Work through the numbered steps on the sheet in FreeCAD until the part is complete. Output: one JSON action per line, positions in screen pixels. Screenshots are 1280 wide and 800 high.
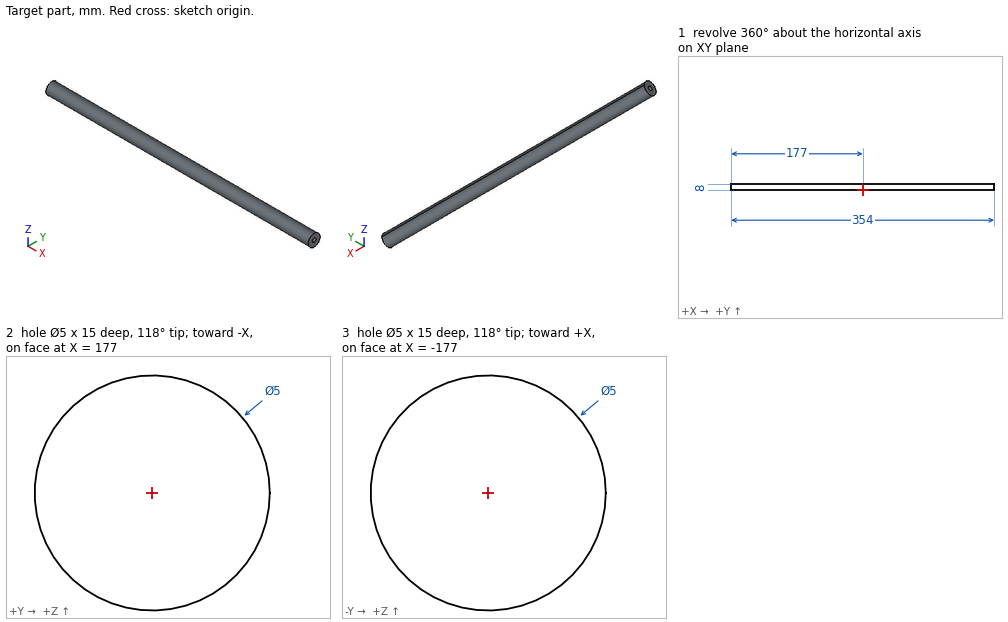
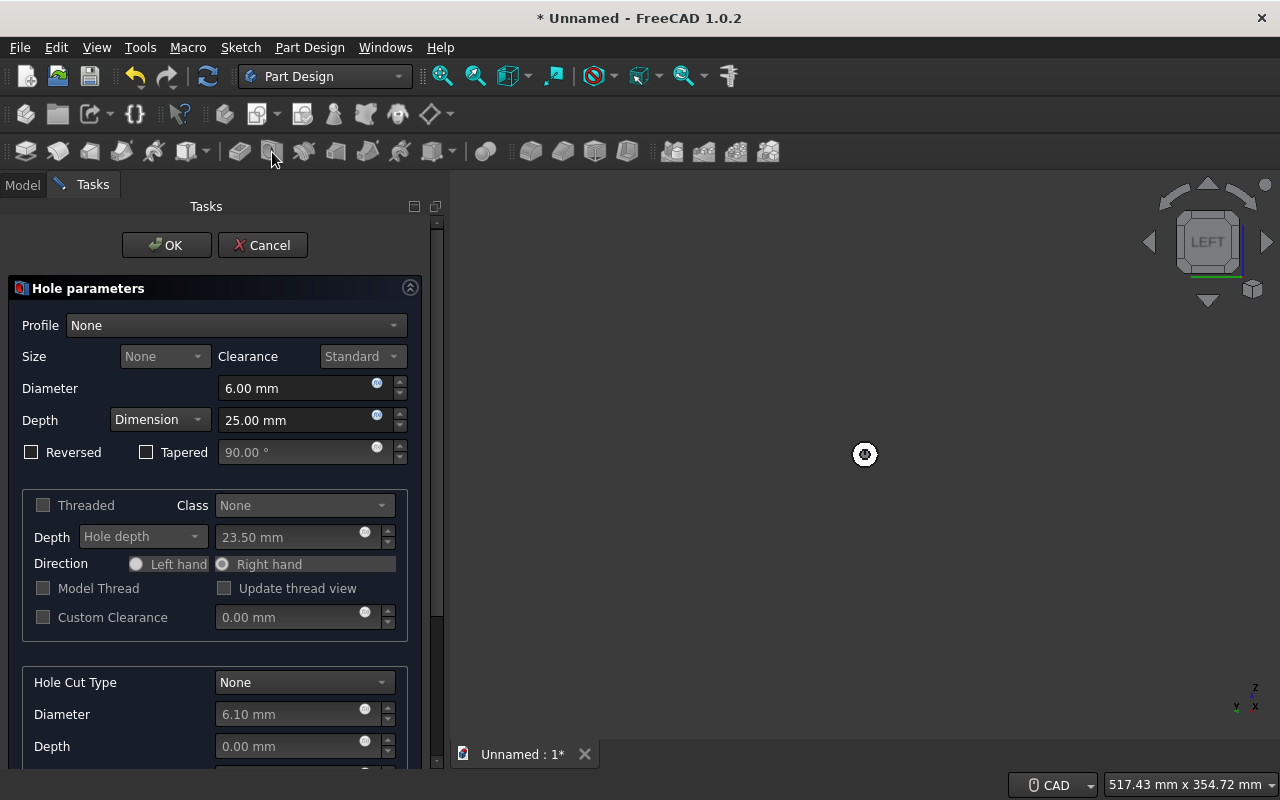
{"action": "triple_click", "coordinate": [305, 388]}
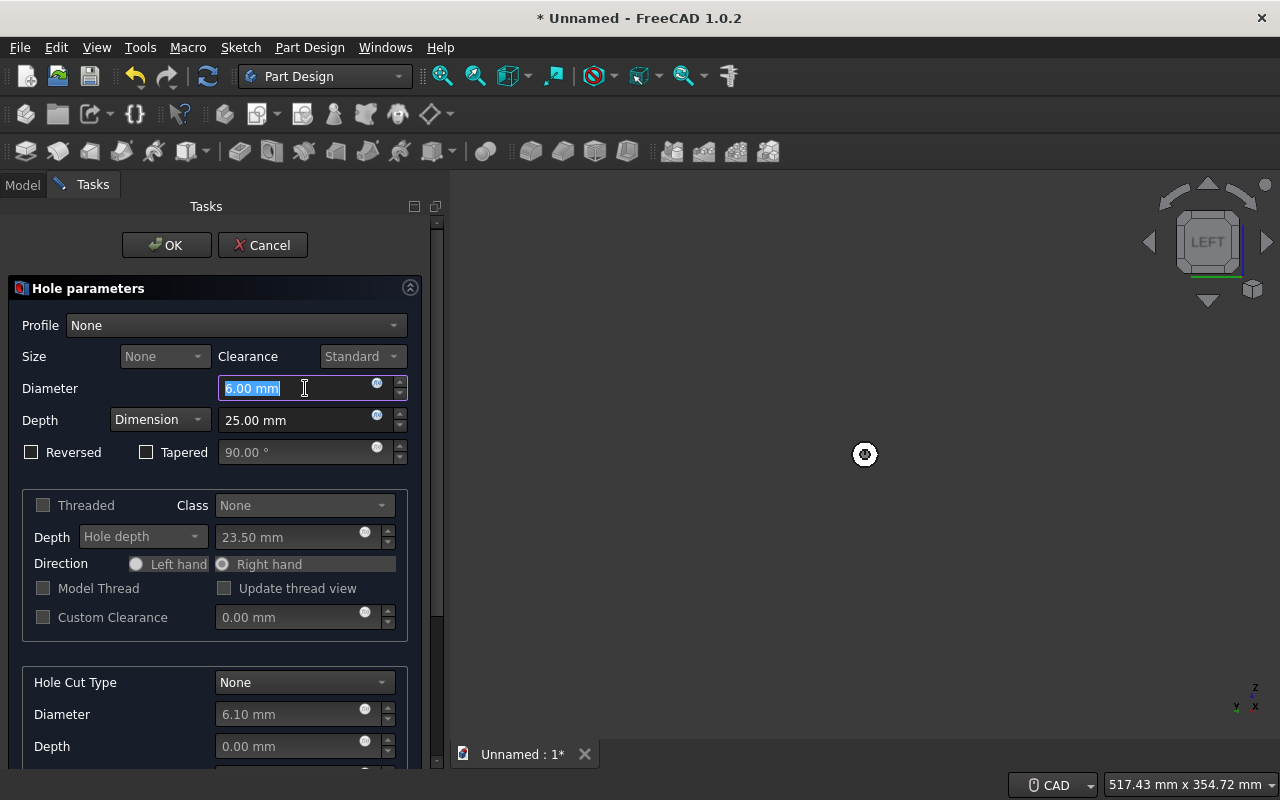
{"action": "type", "text": "5"}
{"action": "key", "text": "Tab"}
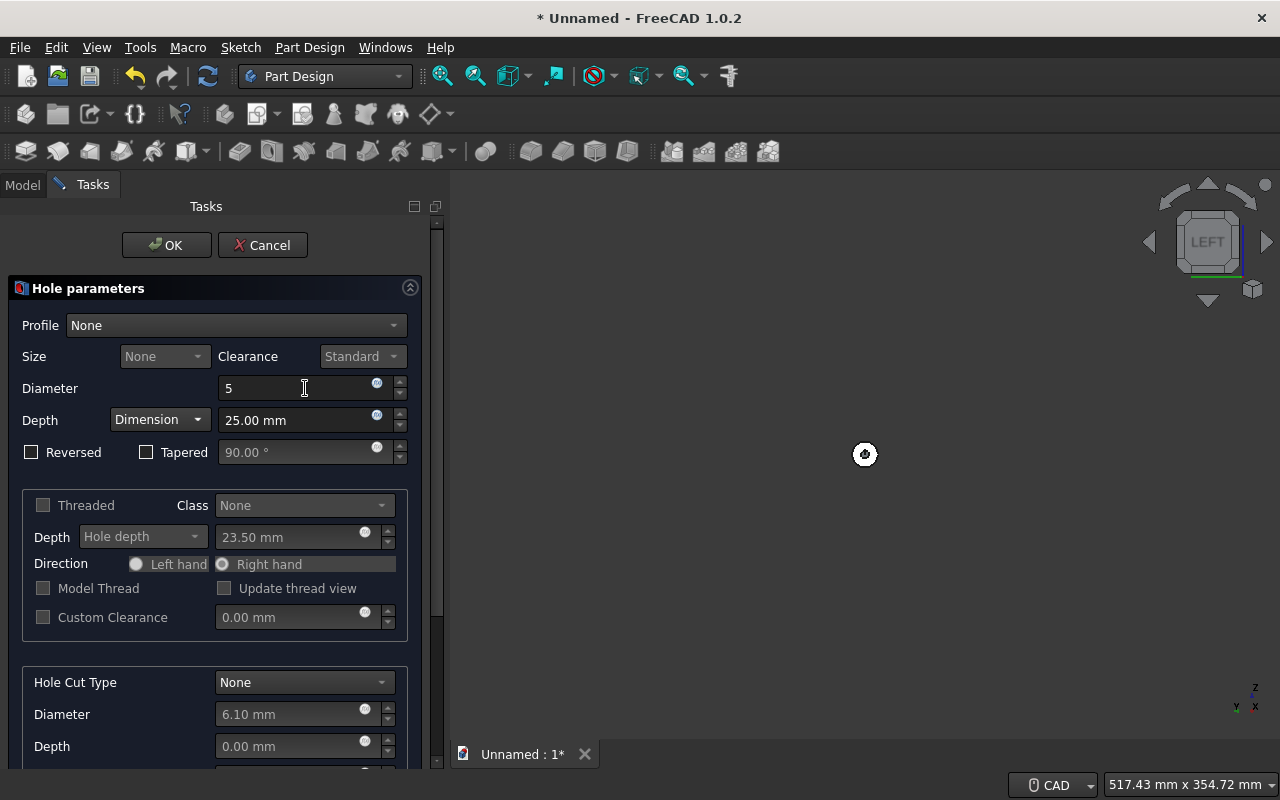
{"action": "triple_click", "coordinate": [305, 420]}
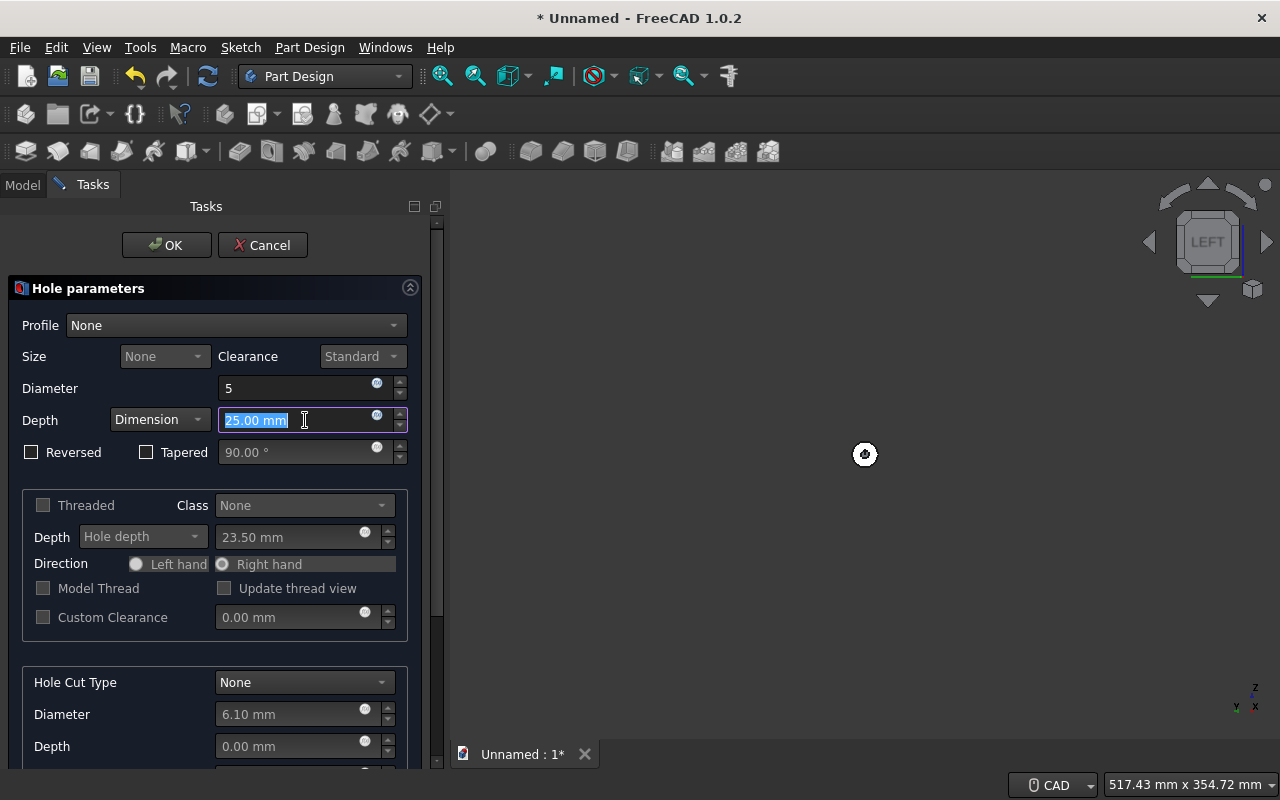
{"action": "type", "text": "15"}
{"action": "key", "text": "Tab"}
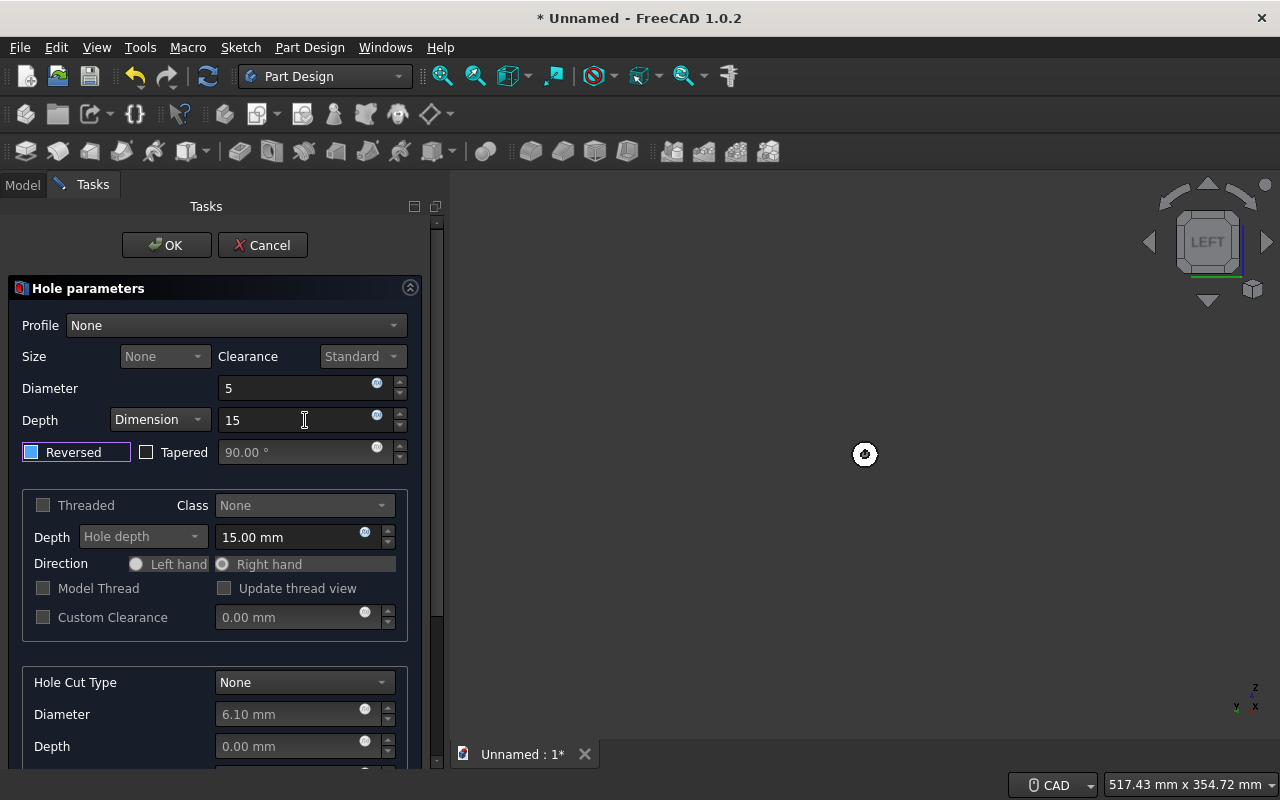
{"action": "left_click", "coordinate": [167, 245]}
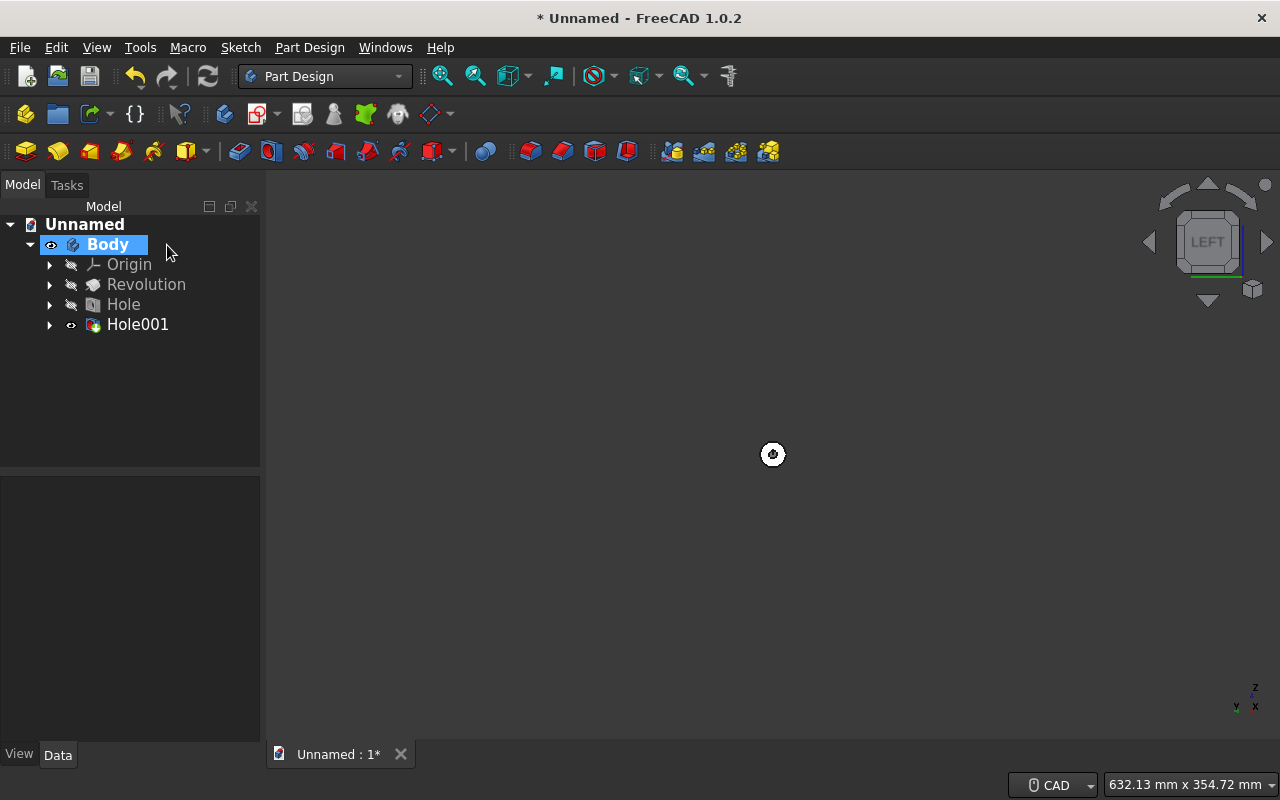
{"action": "key", "text": "0"}